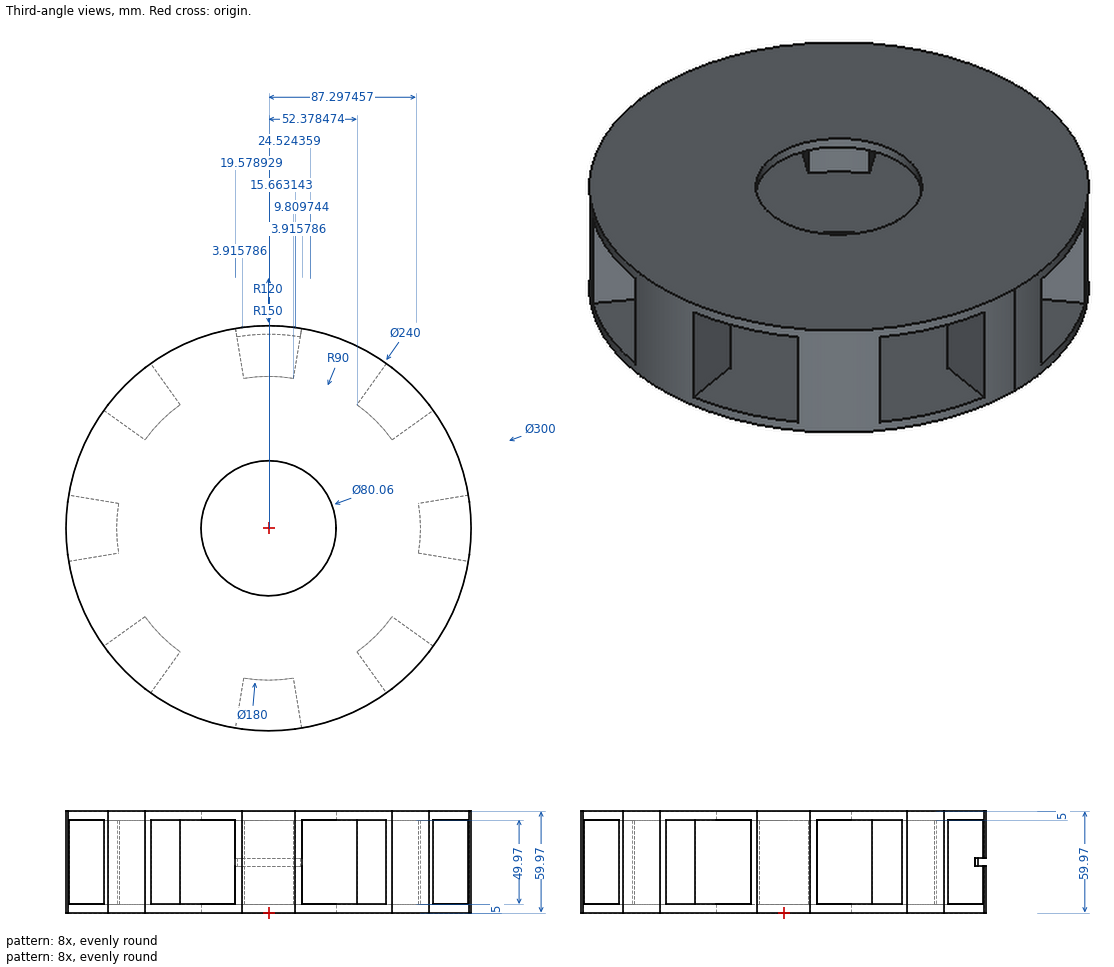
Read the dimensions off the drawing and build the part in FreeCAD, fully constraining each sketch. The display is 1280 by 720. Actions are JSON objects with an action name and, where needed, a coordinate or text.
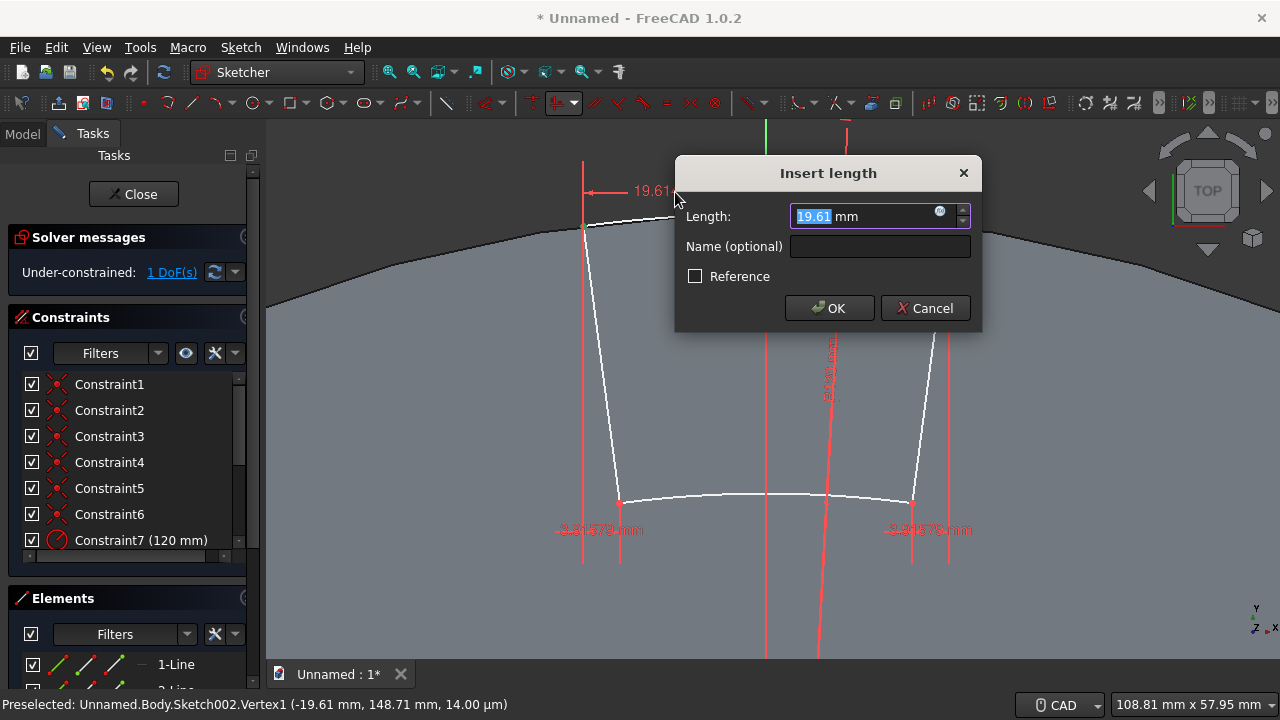
{"action": "type", "text": "19.578929"}
{"action": "key", "text": "Return"}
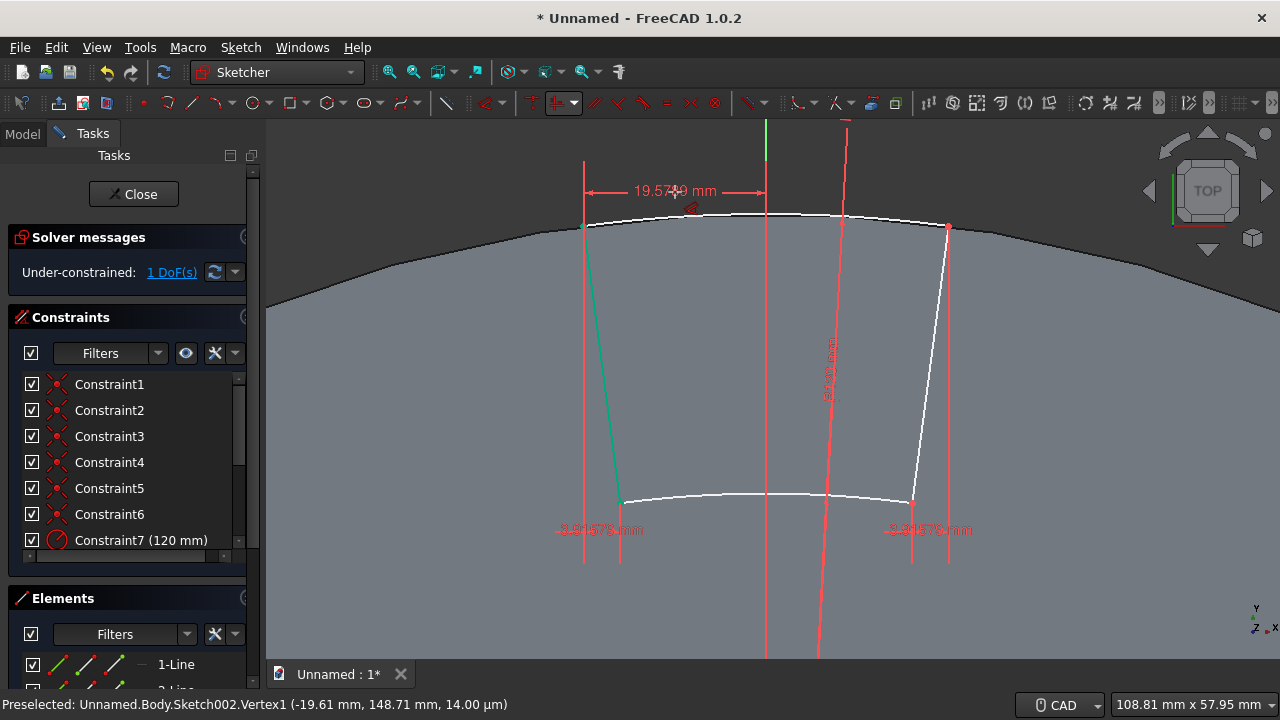
{"action": "left_click", "coordinate": [912, 503]}
{"action": "left_click", "coordinate": [839, 469]}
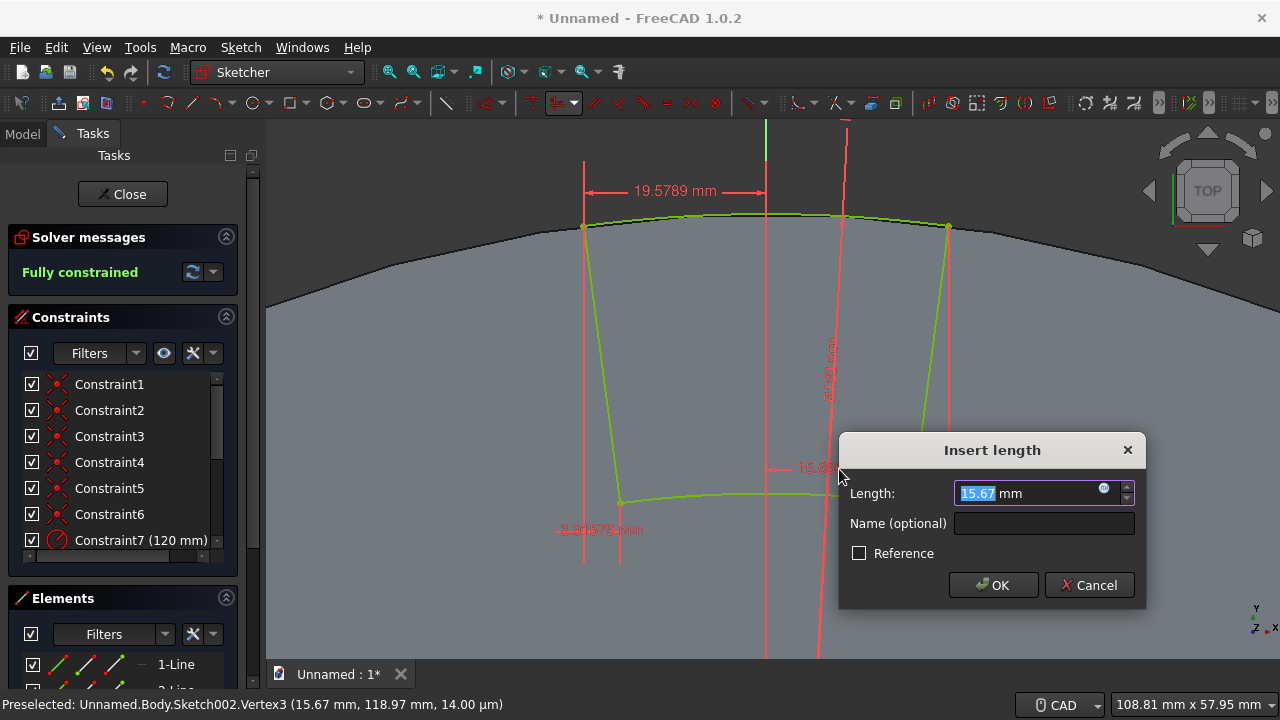
{"action": "type", "text": "15.663143"}
{"action": "key", "text": "Return"}
{"action": "key", "text": "Escape"}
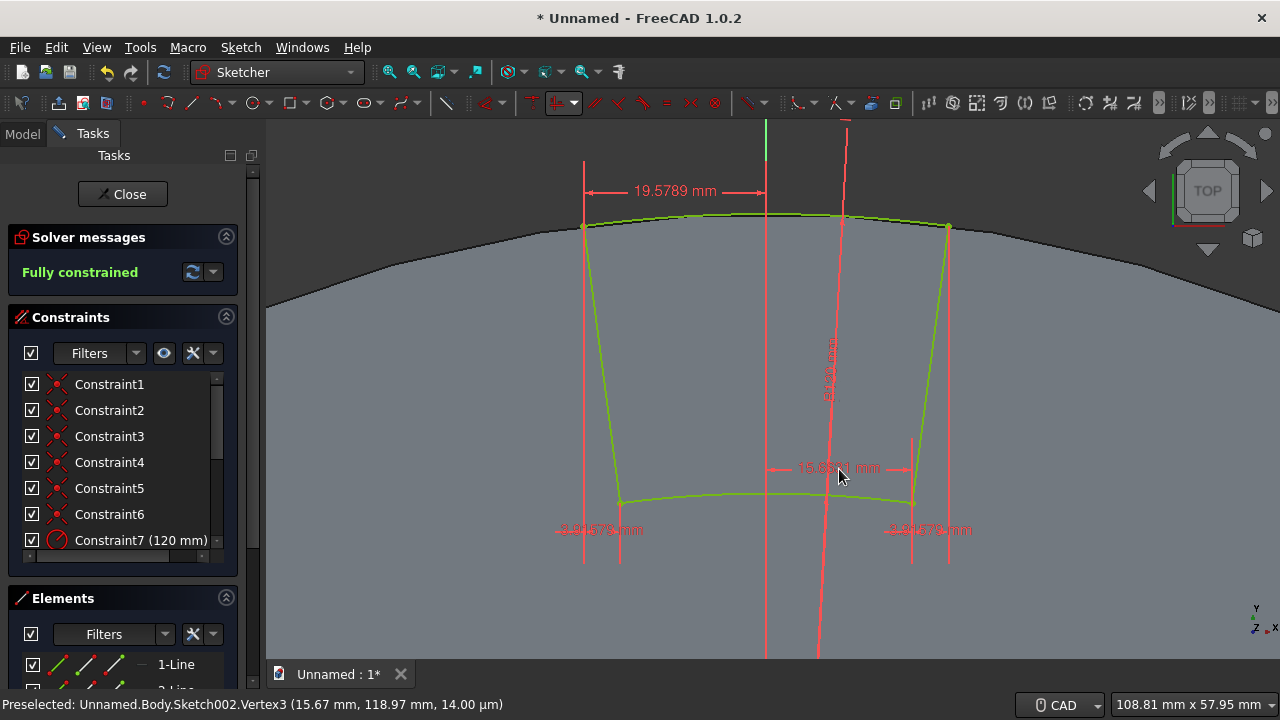
{"action": "left_click", "coordinate": [123, 194]}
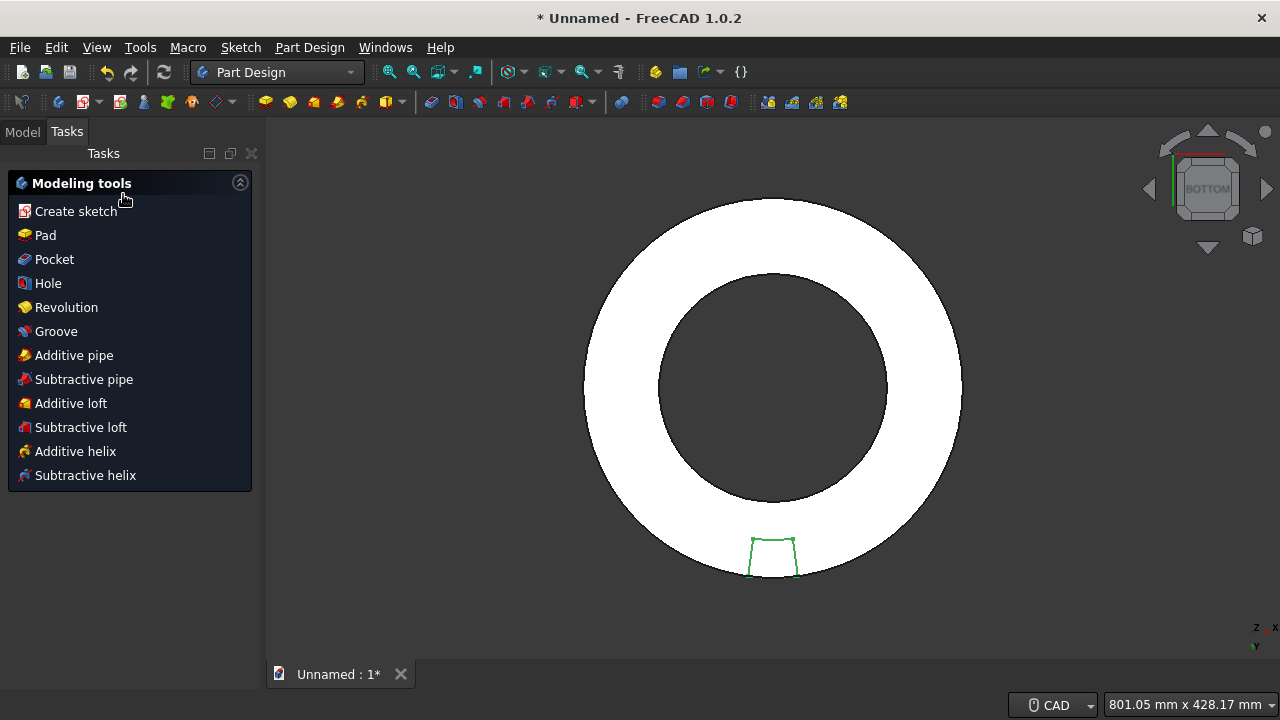
{"action": "left_click", "coordinate": [432, 102]}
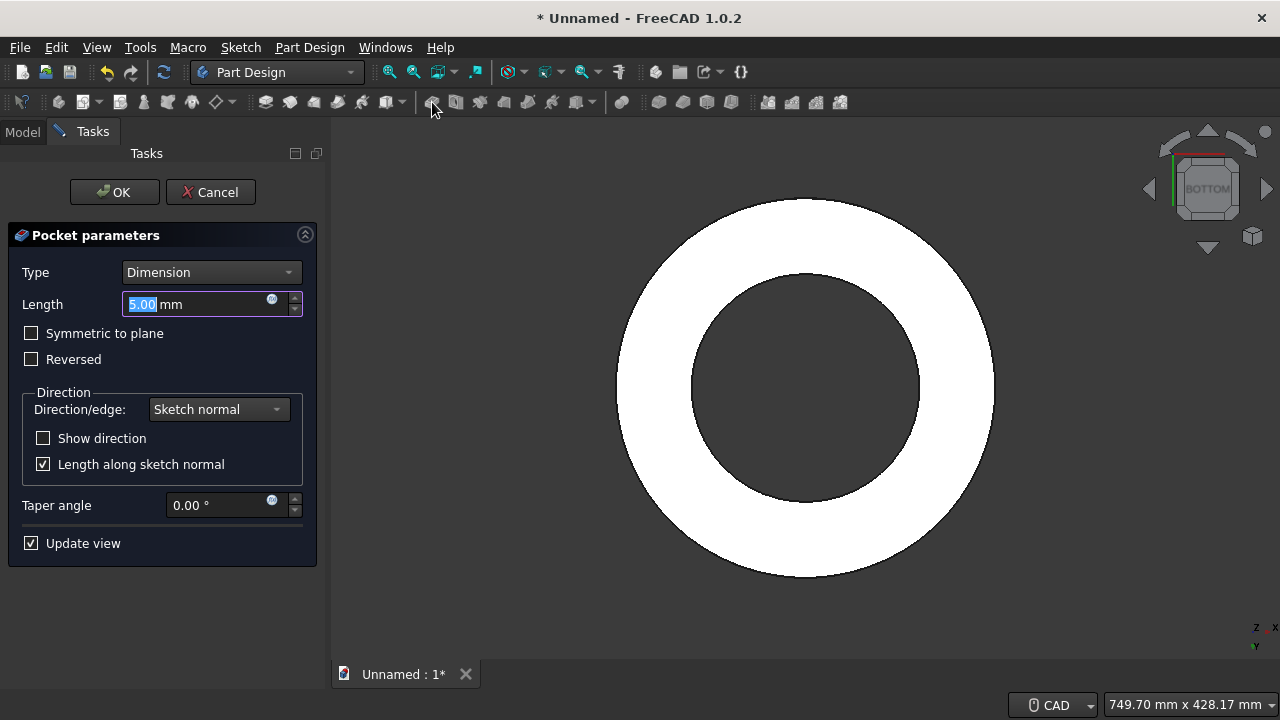
{"action": "type", "text": "59.97"}
{"action": "key", "text": "Tab"}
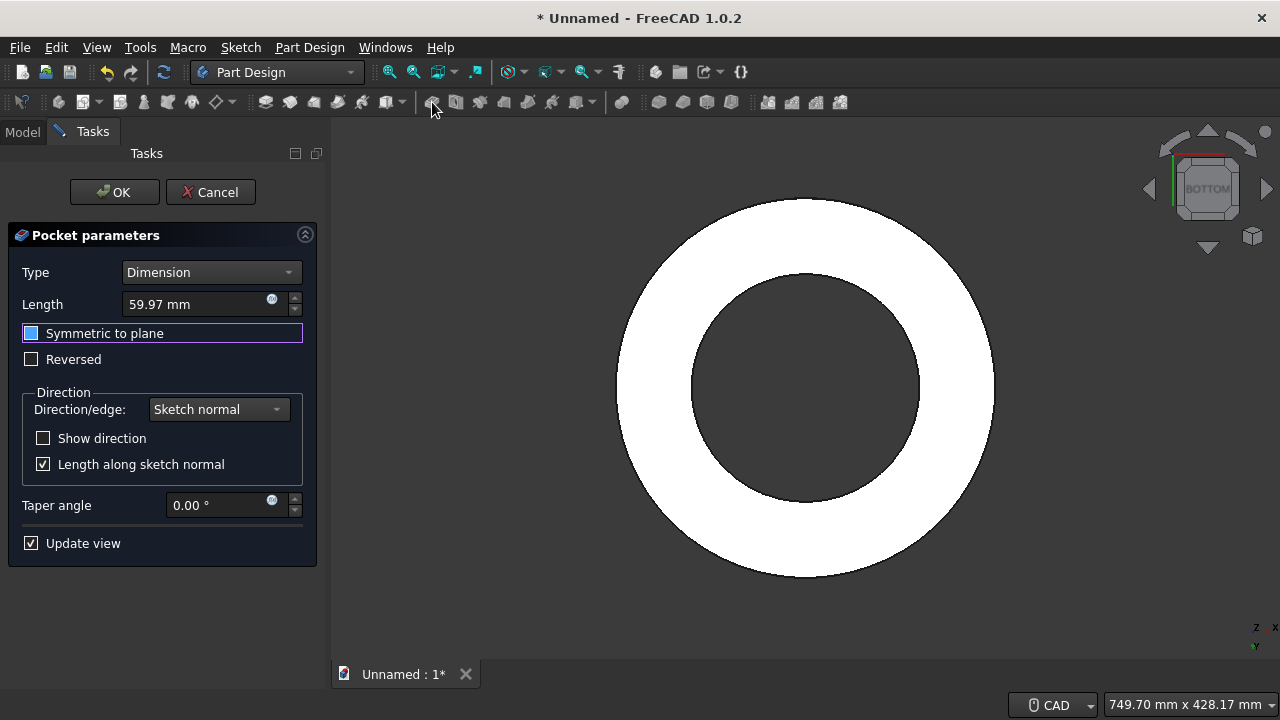
{"action": "left_click", "coordinate": [30, 359]}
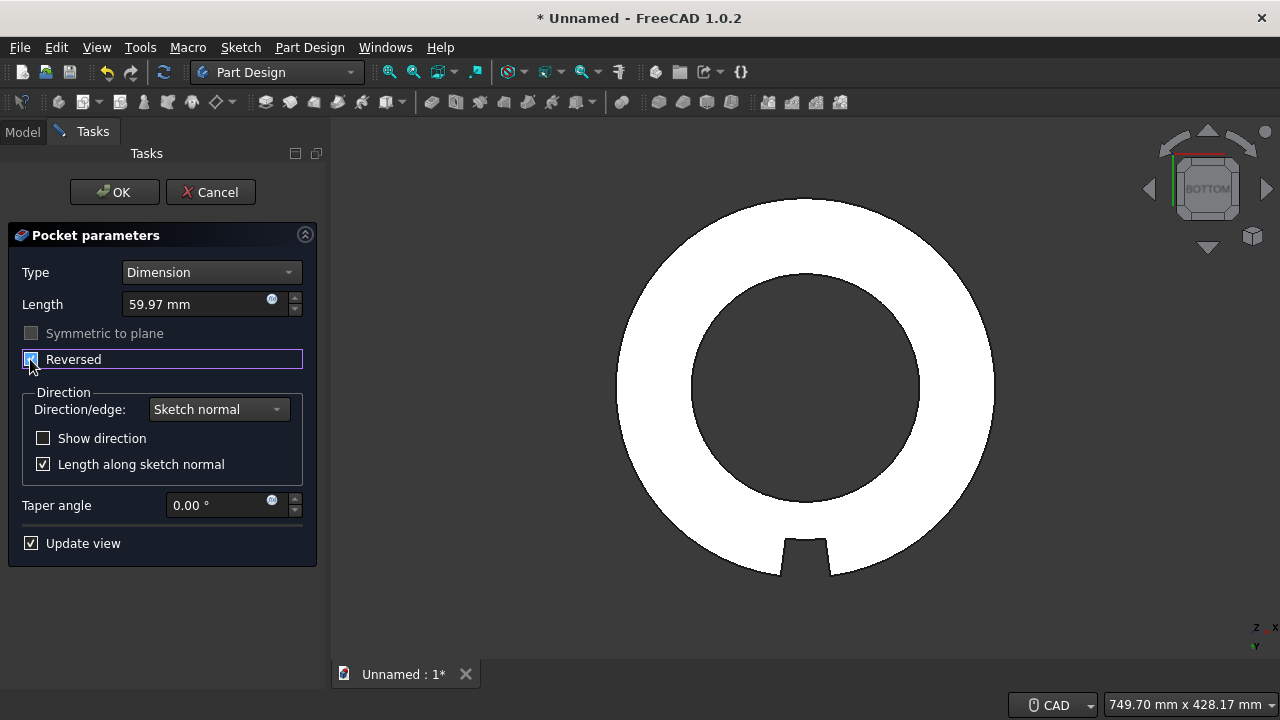
{"action": "left_click", "coordinate": [115, 192]}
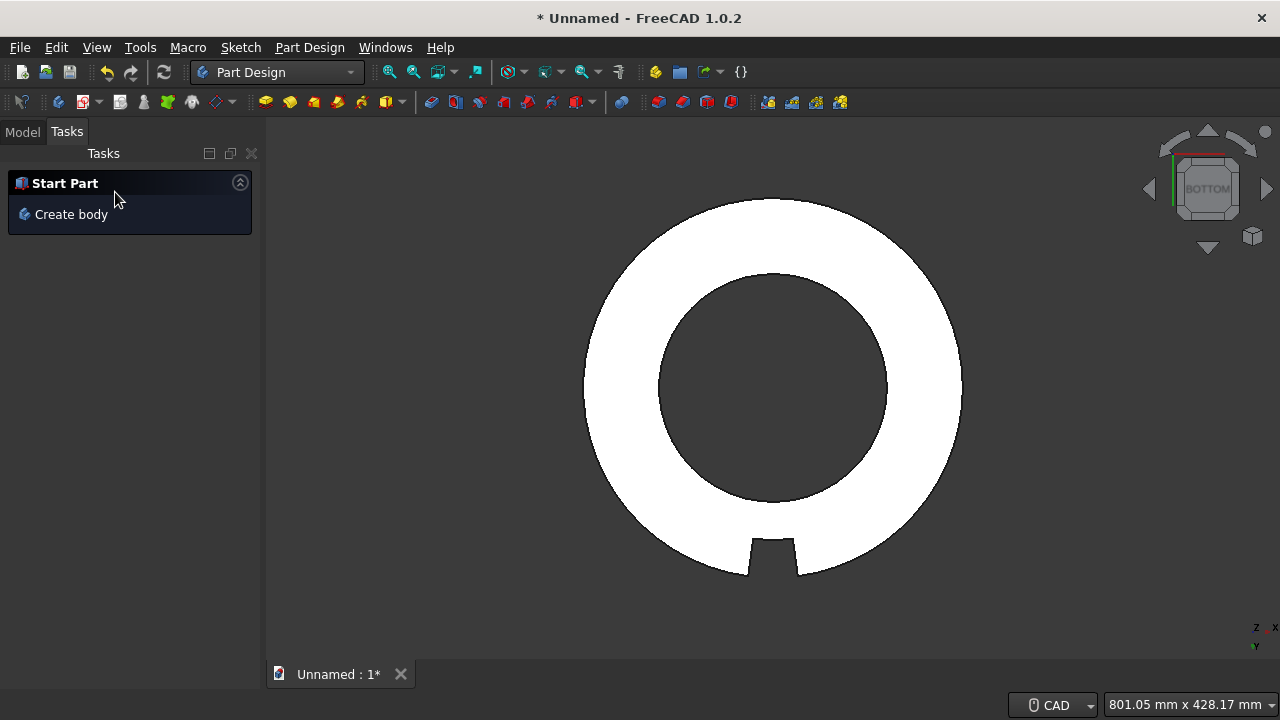
{"action": "left_click", "coordinate": [23, 131]}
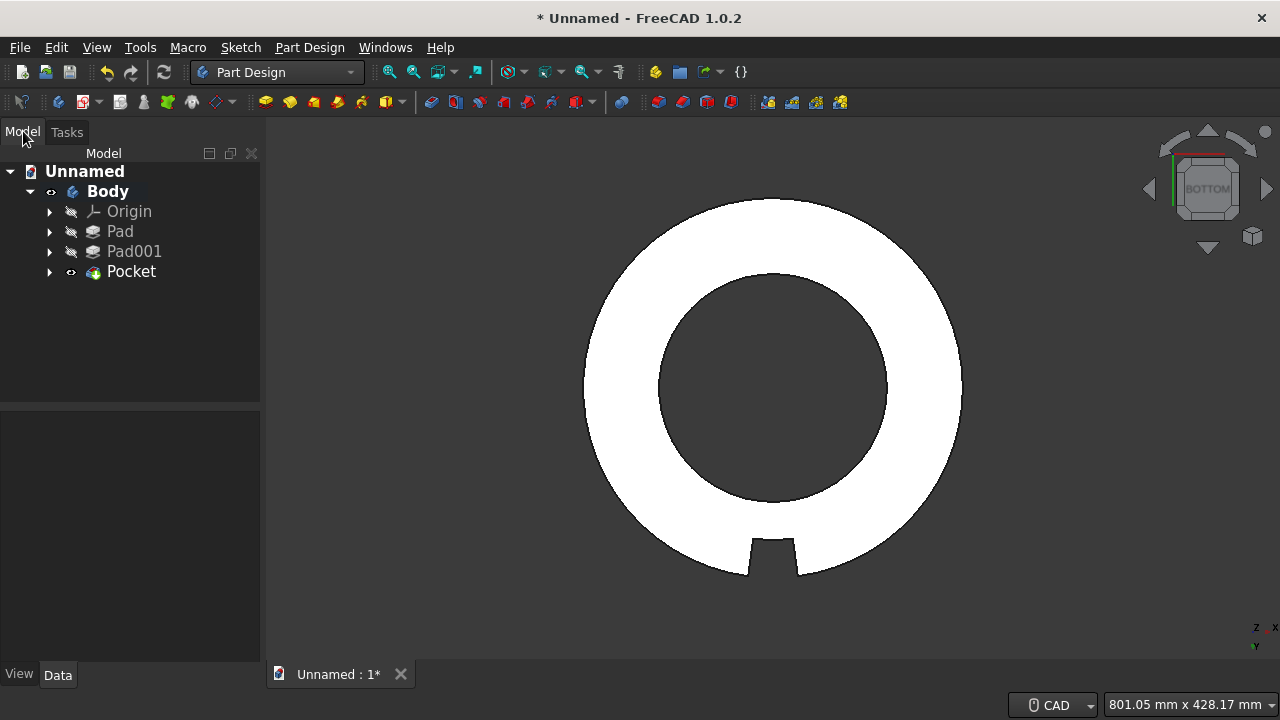
{"action": "left_click", "coordinate": [116, 272]}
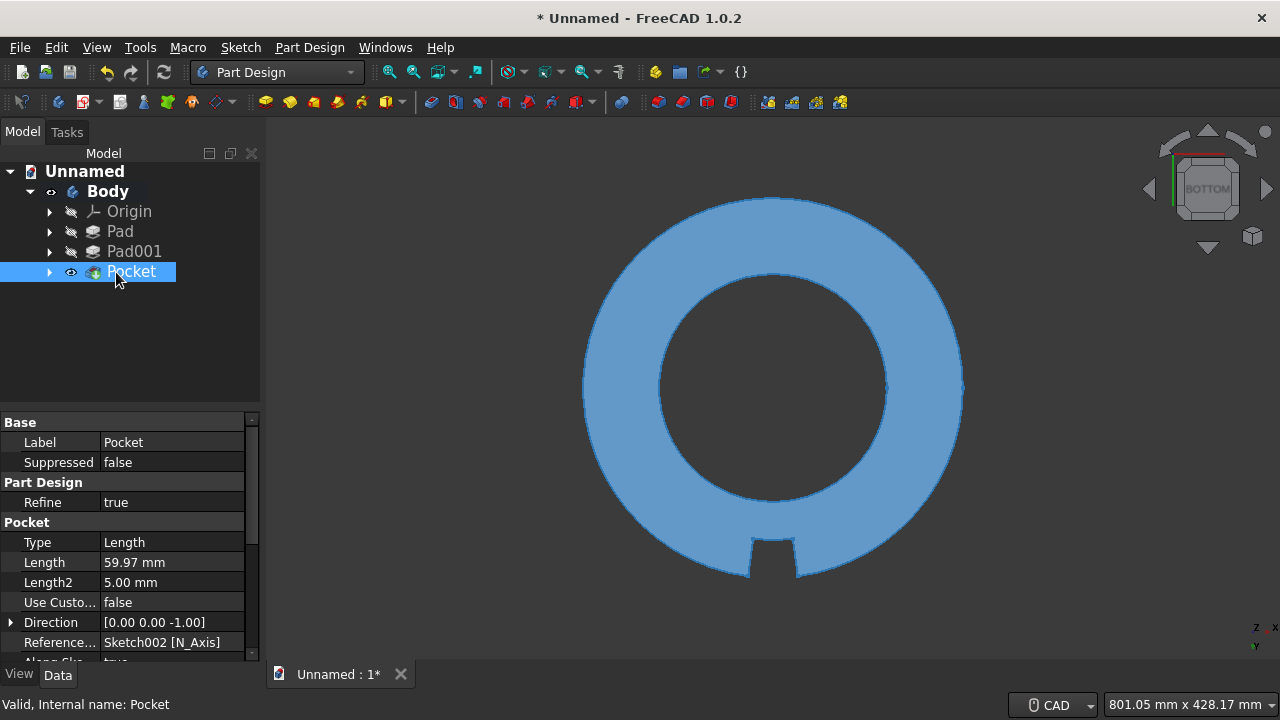
{"action": "left_click", "coordinate": [816, 102]}